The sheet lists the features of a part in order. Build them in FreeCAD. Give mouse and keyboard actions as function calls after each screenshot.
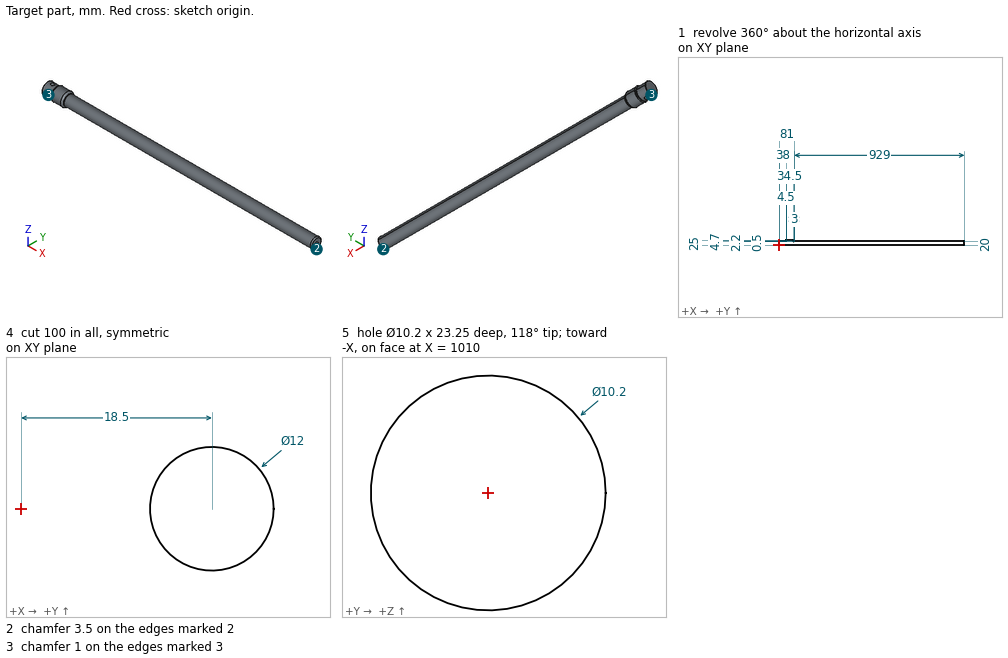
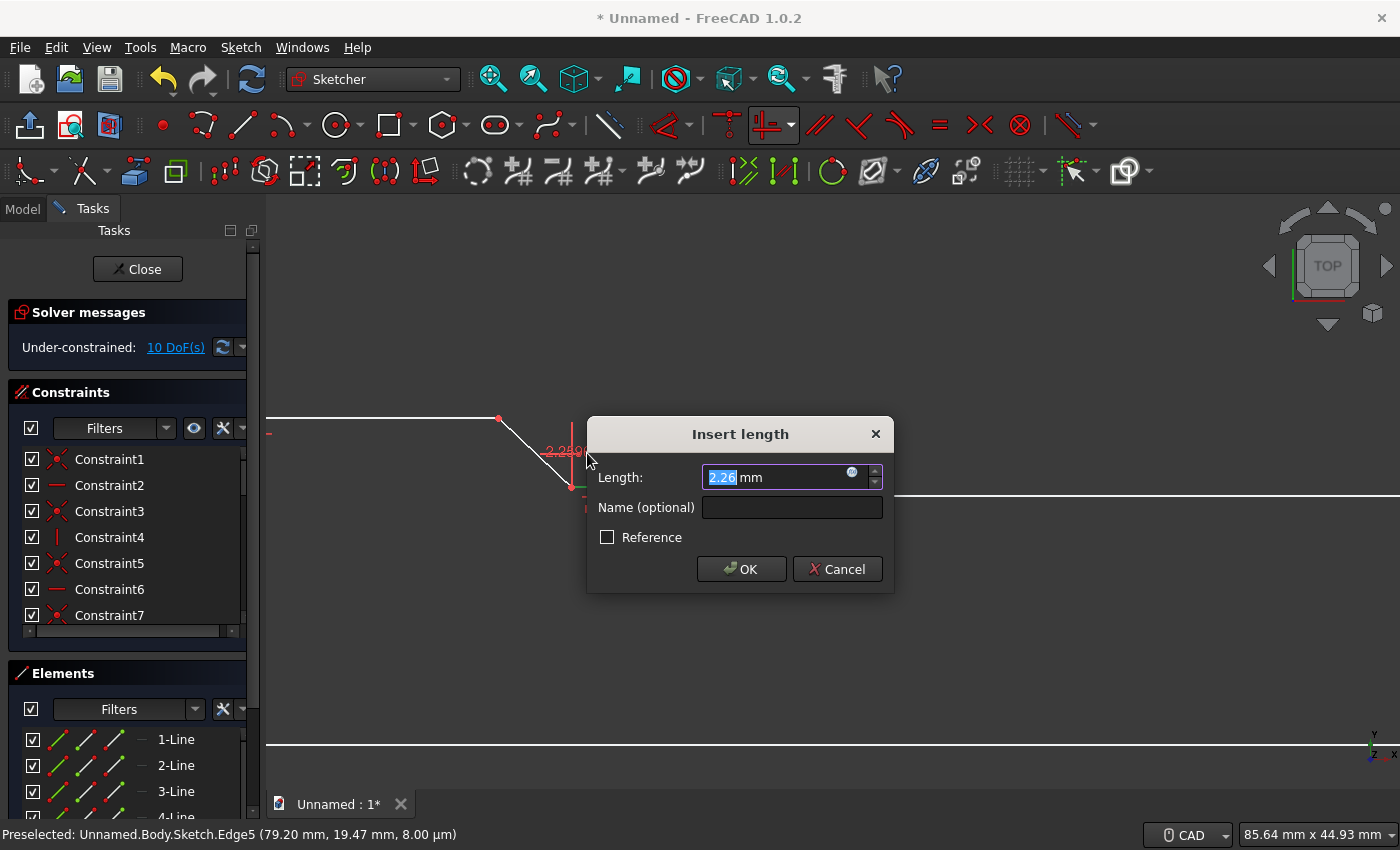
text(3)
key(Return)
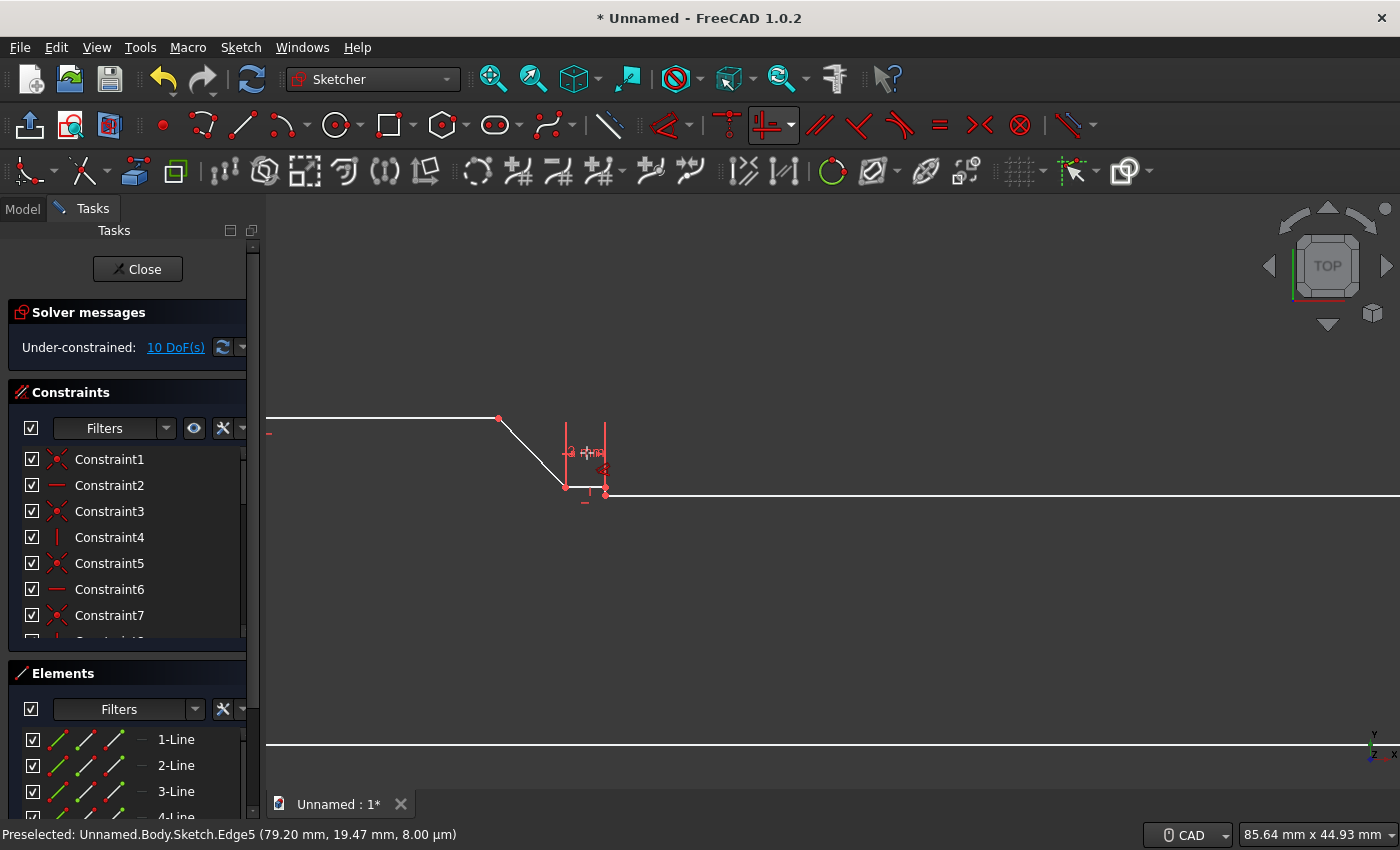
scroll(478, 487, down, 15)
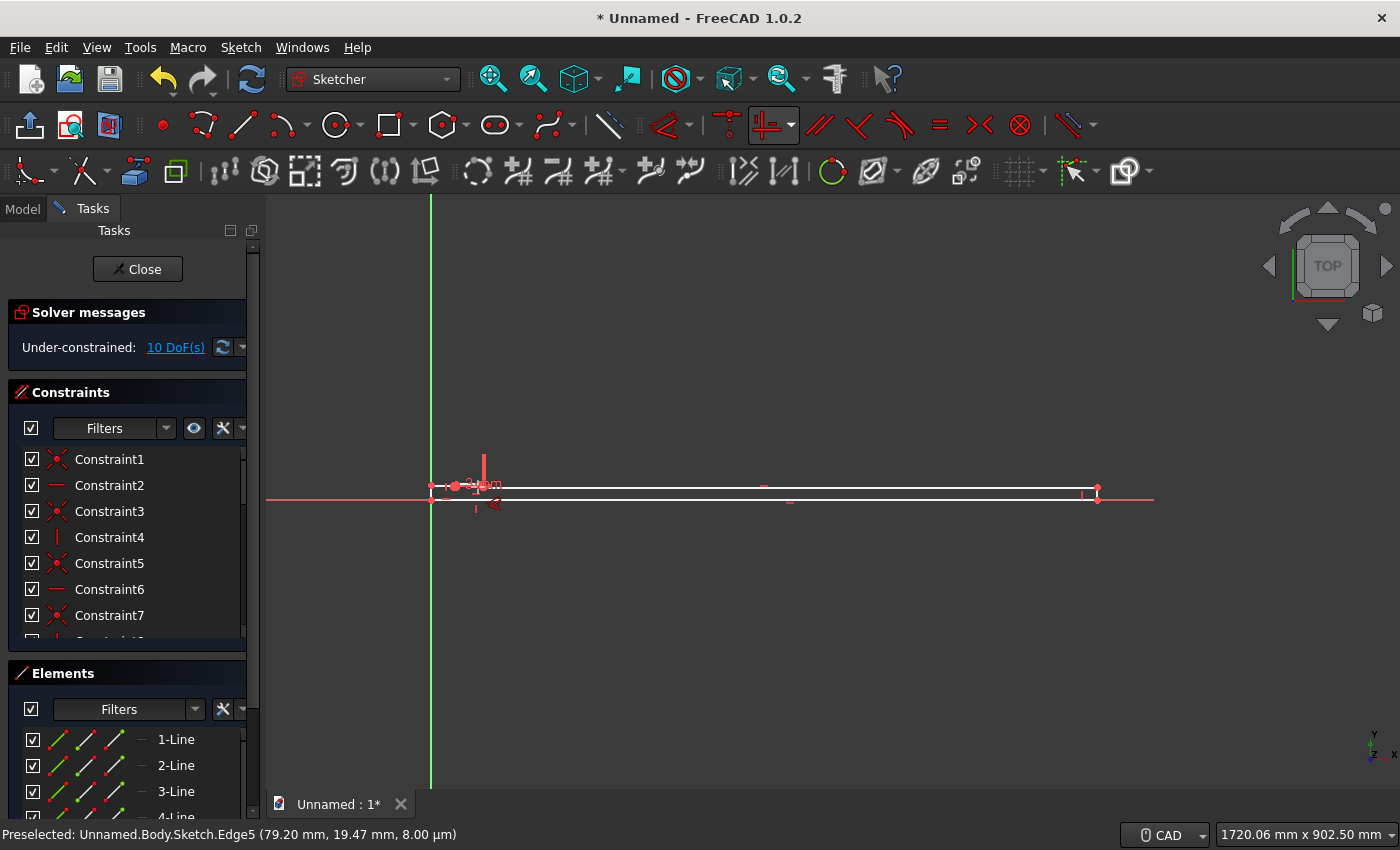
scroll(1097, 497, up, 7)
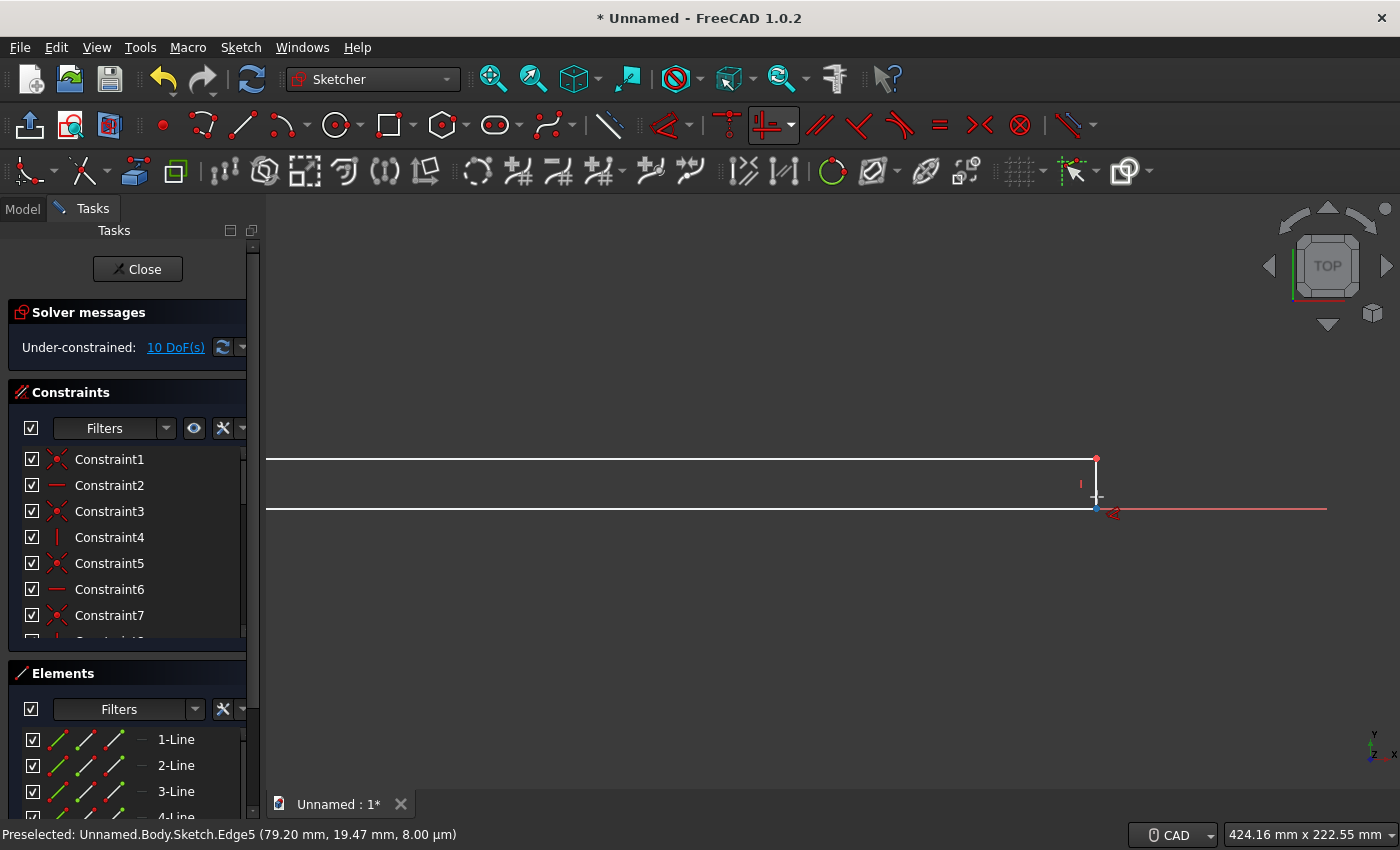
click(1096, 494)
click(1130, 484)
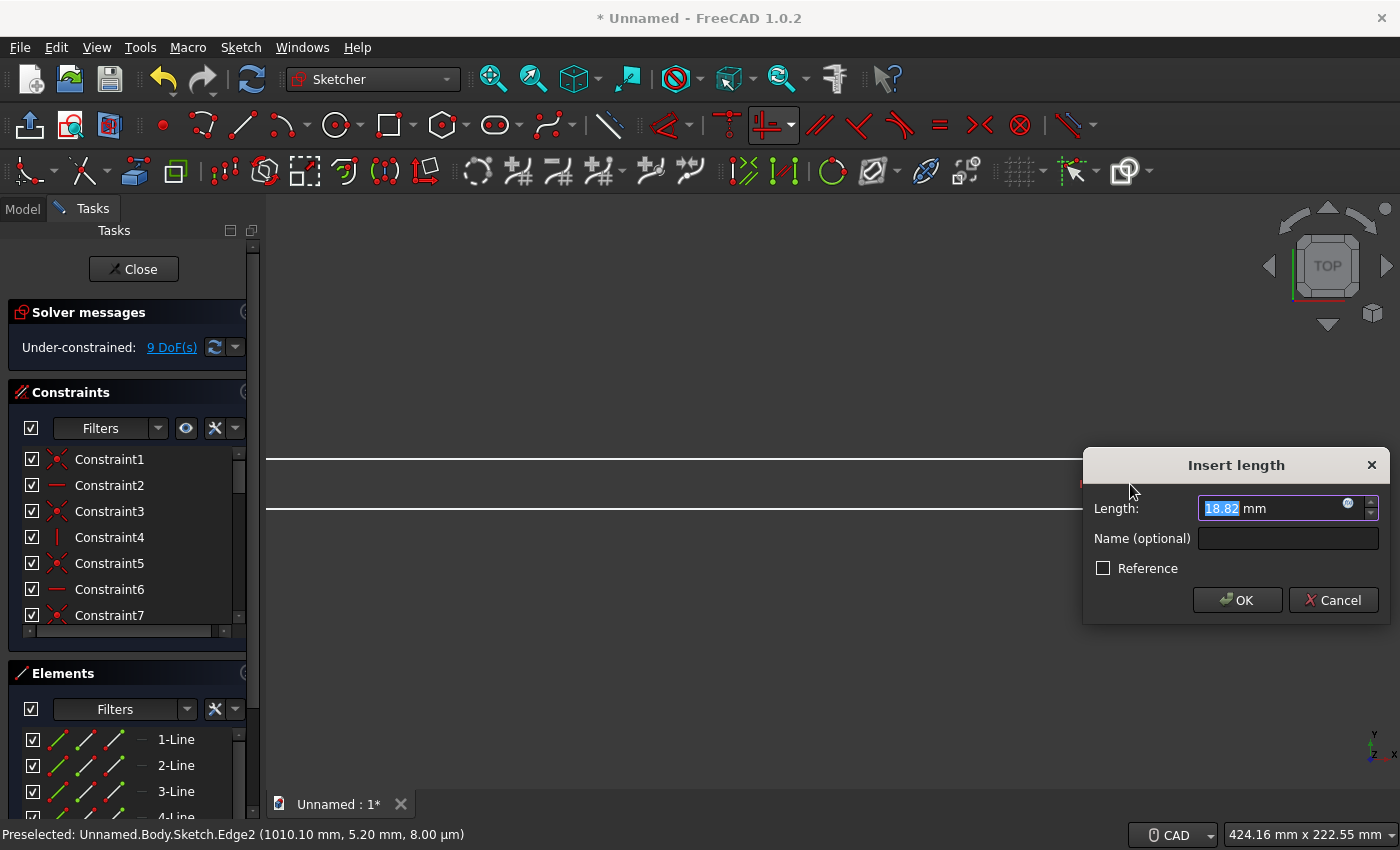
text(20)
key(Return)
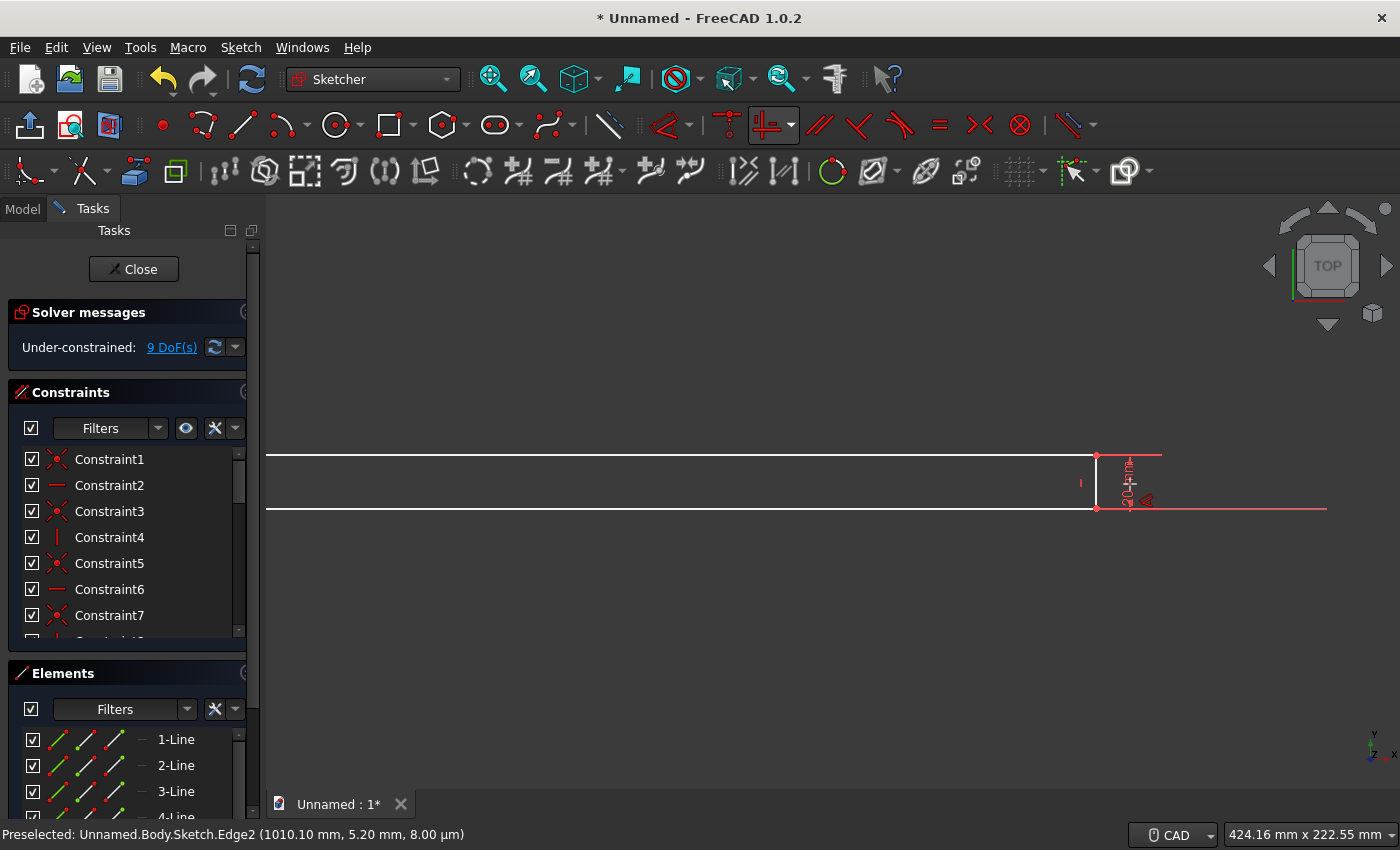
scroll(1098, 497, down, 7)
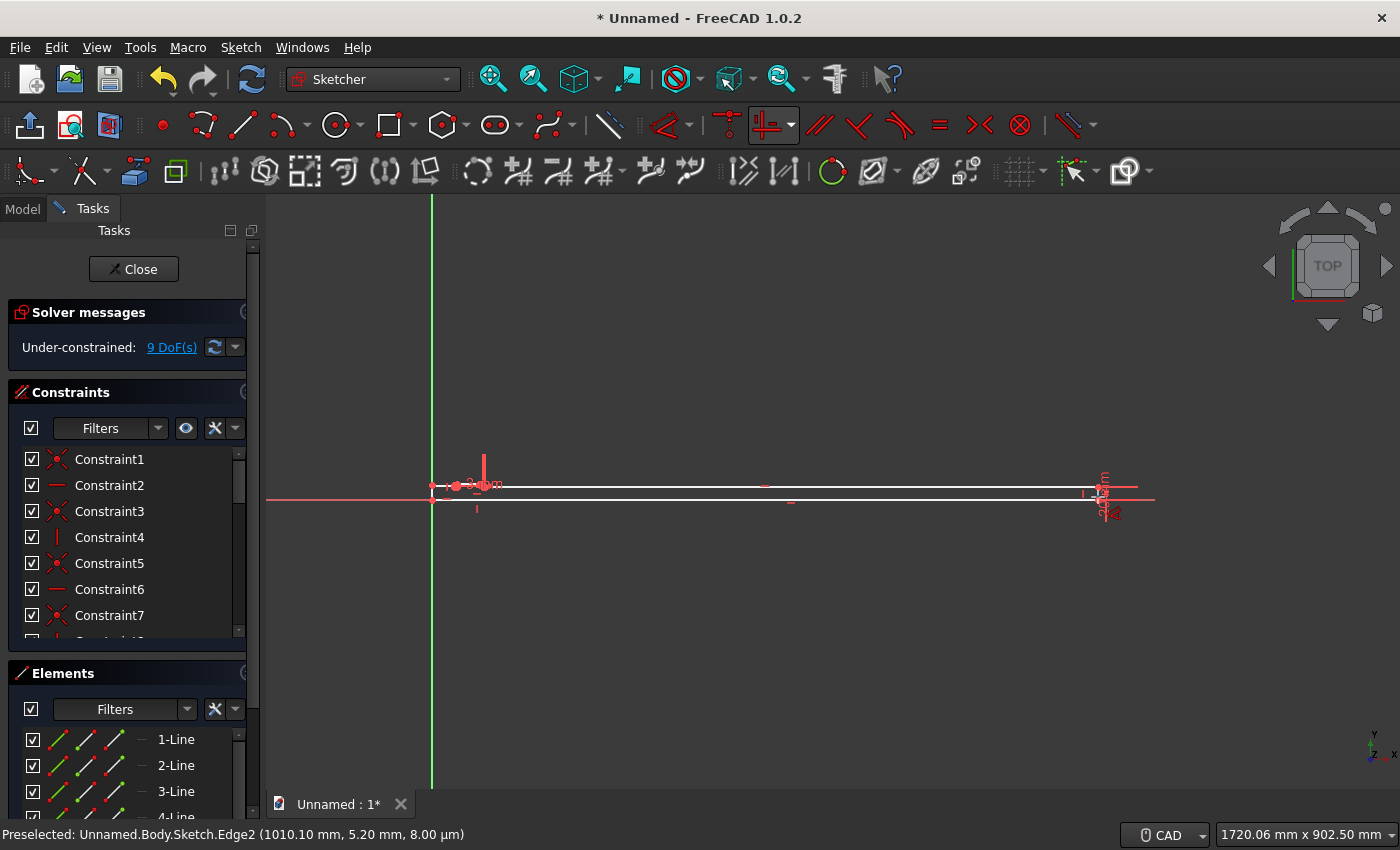
click(914, 487)
click(792, 453)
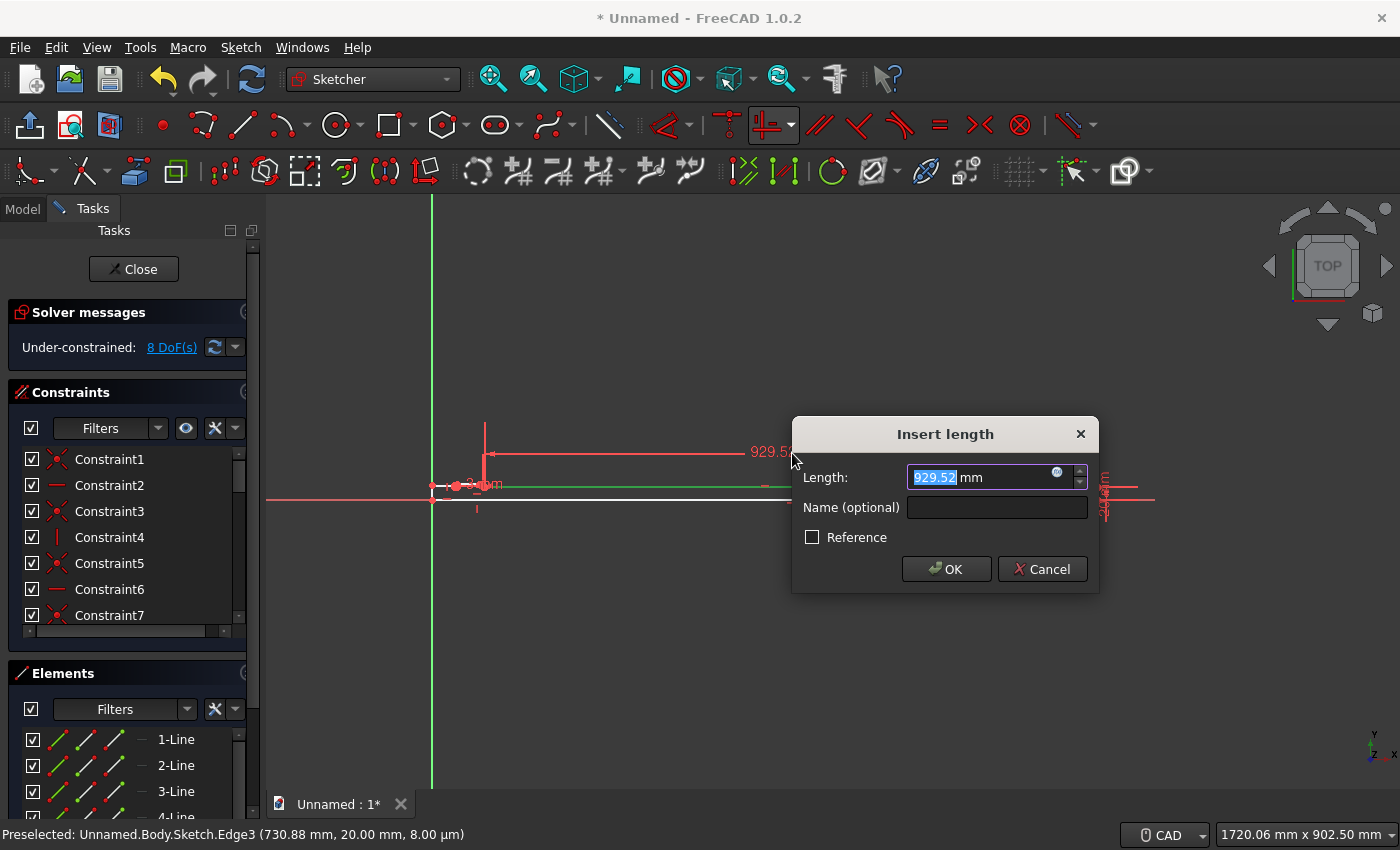
text(929)
key(Return)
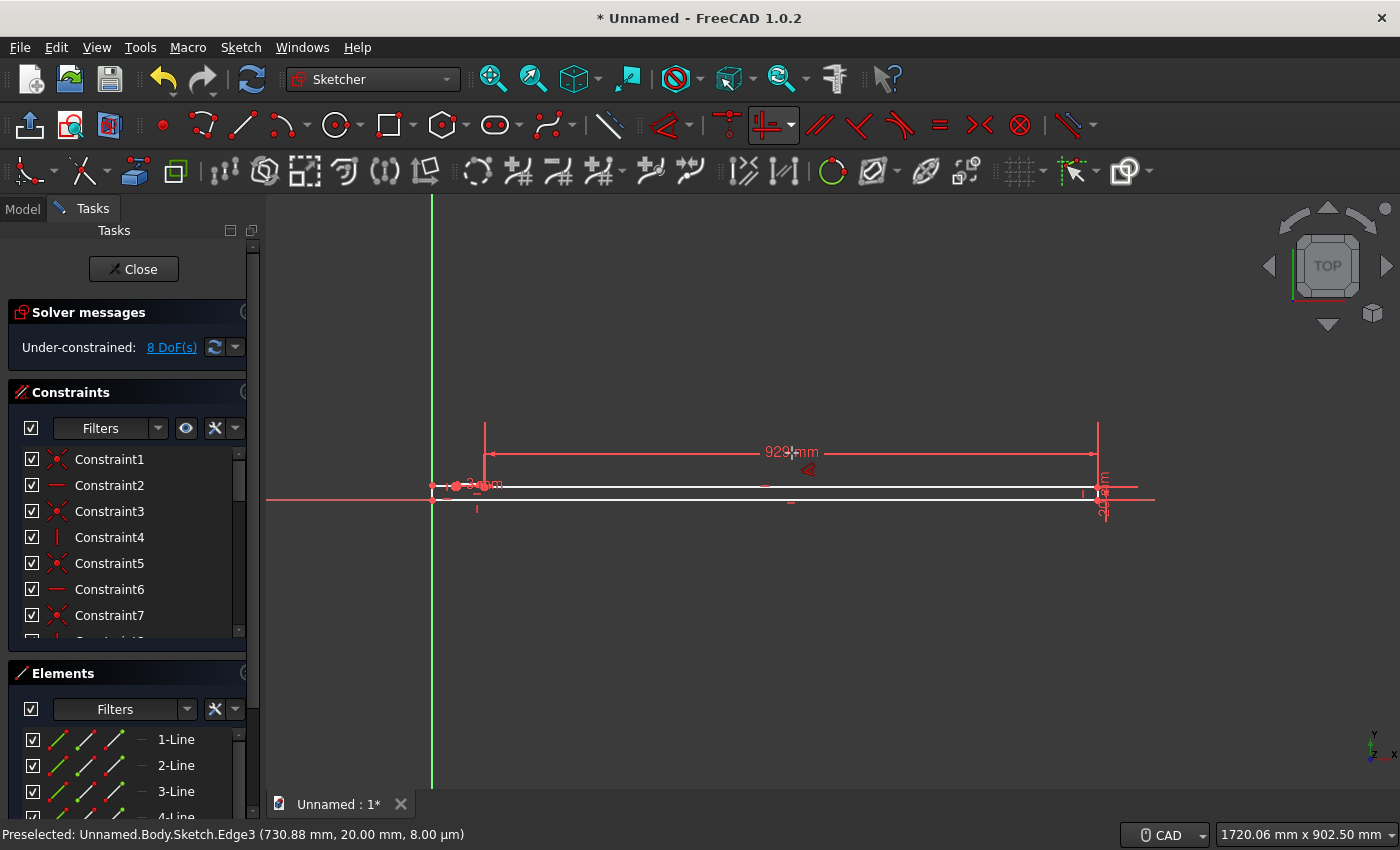
scroll(485, 487, up, 24)